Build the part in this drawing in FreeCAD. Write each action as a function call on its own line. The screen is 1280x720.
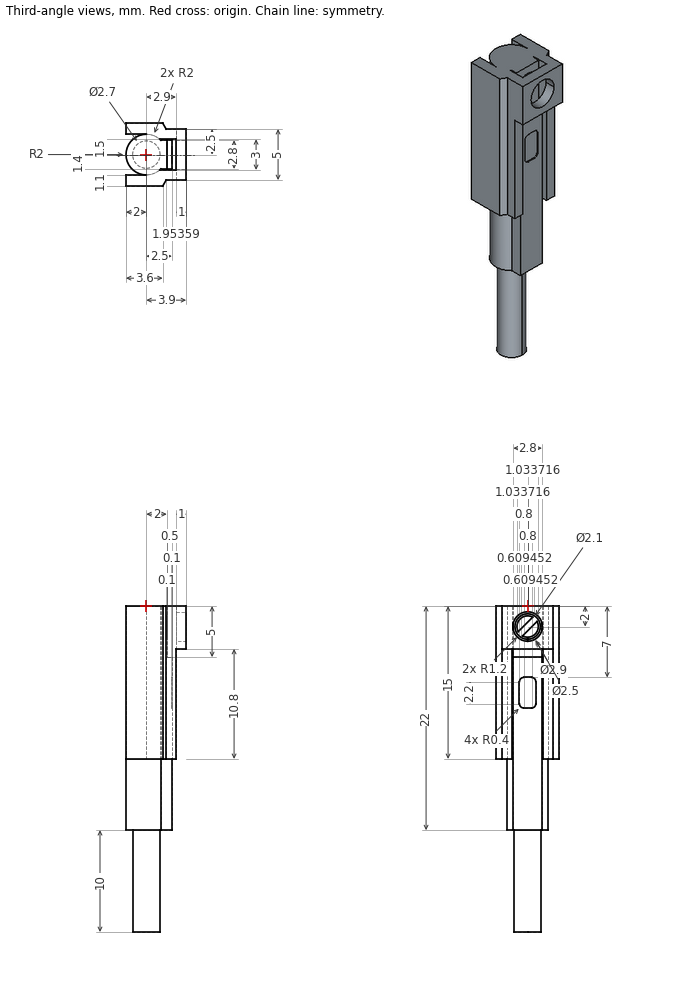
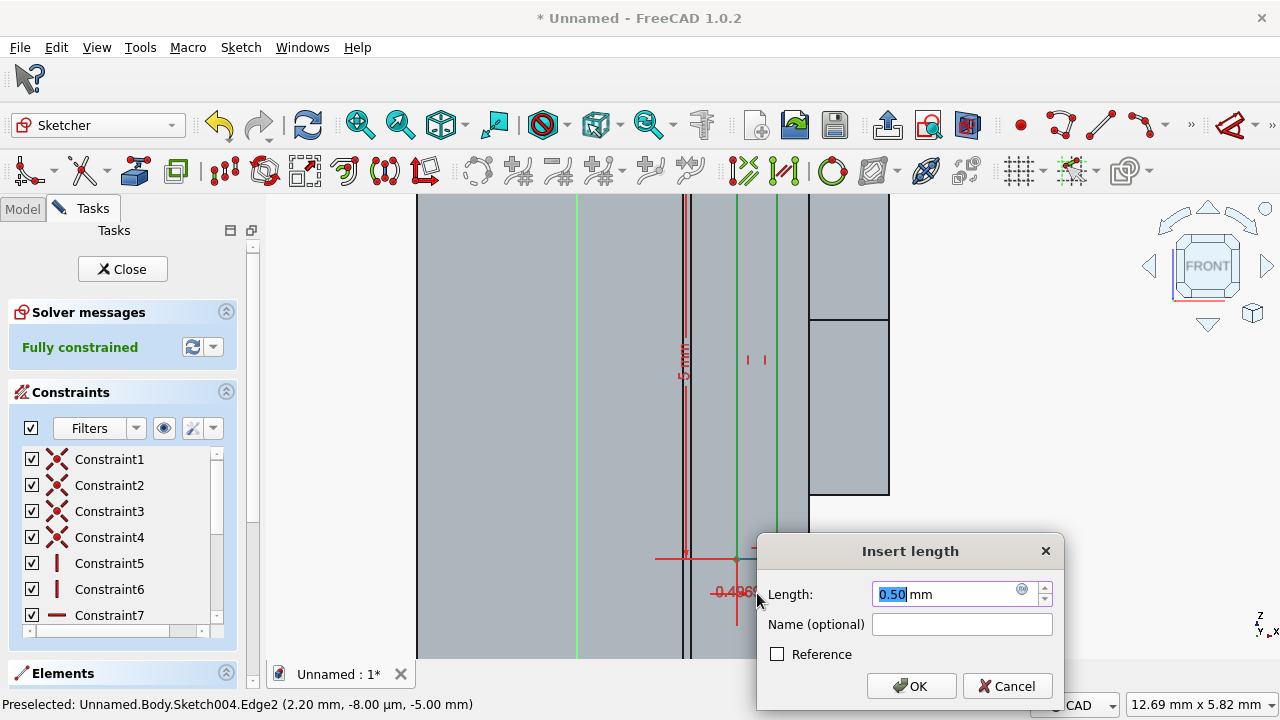
text(0.5)
key(Return)
key(Escape)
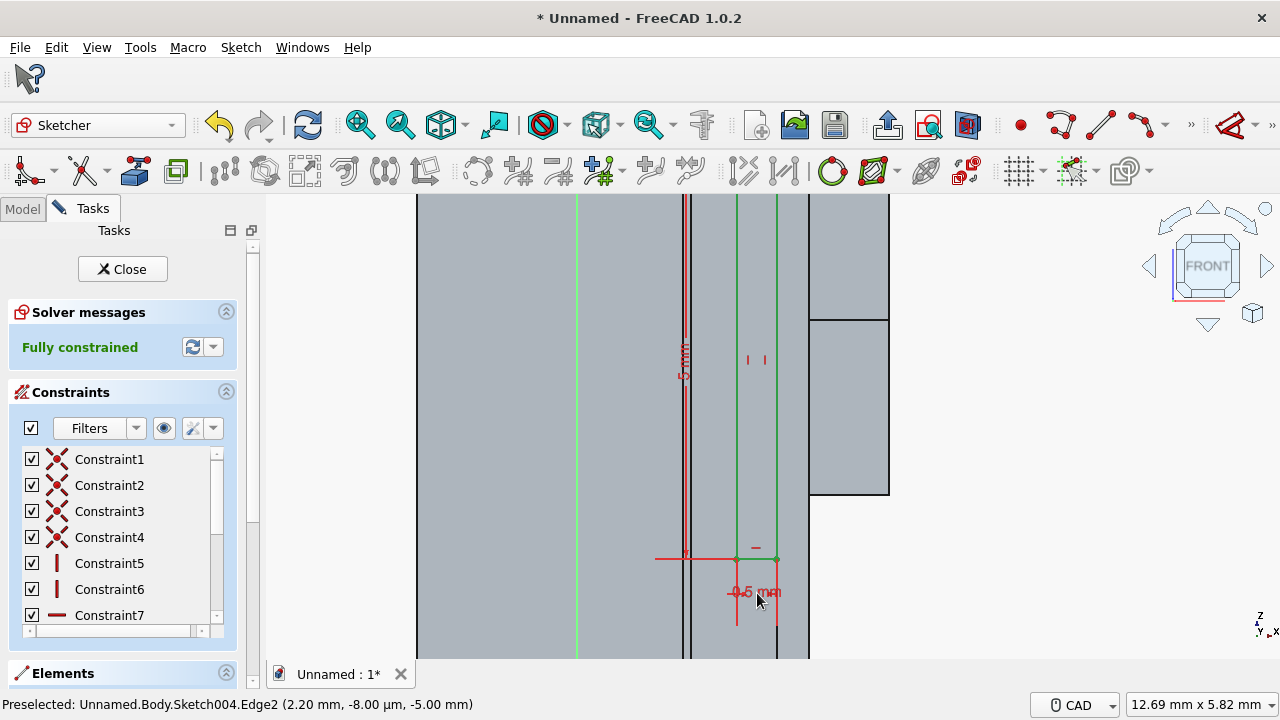
click(123, 269)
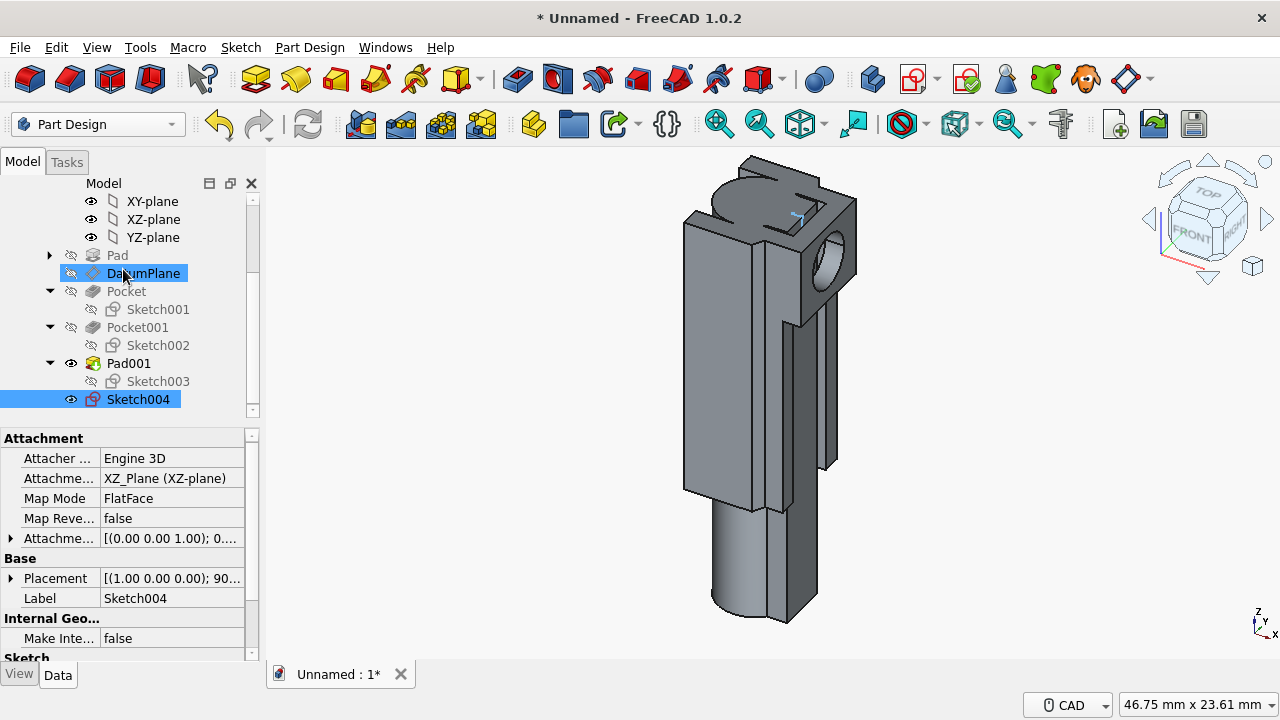
click(518, 80)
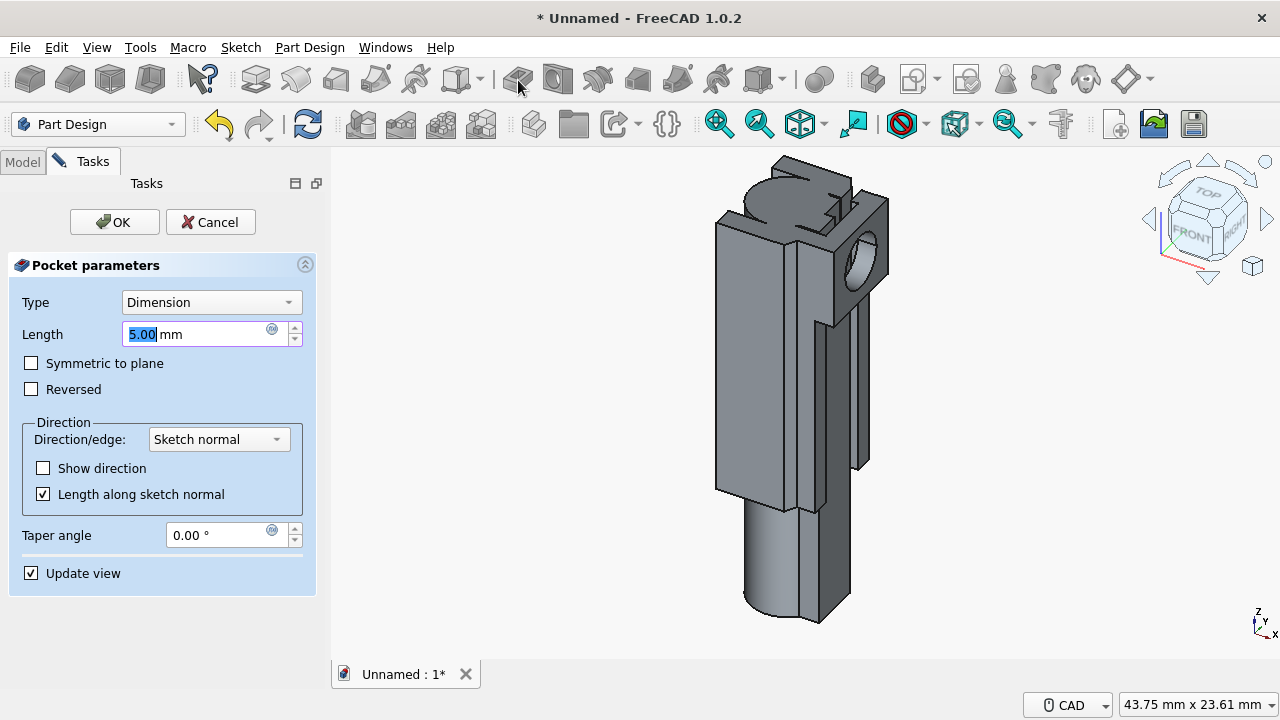
text(2.8)
key(Tab)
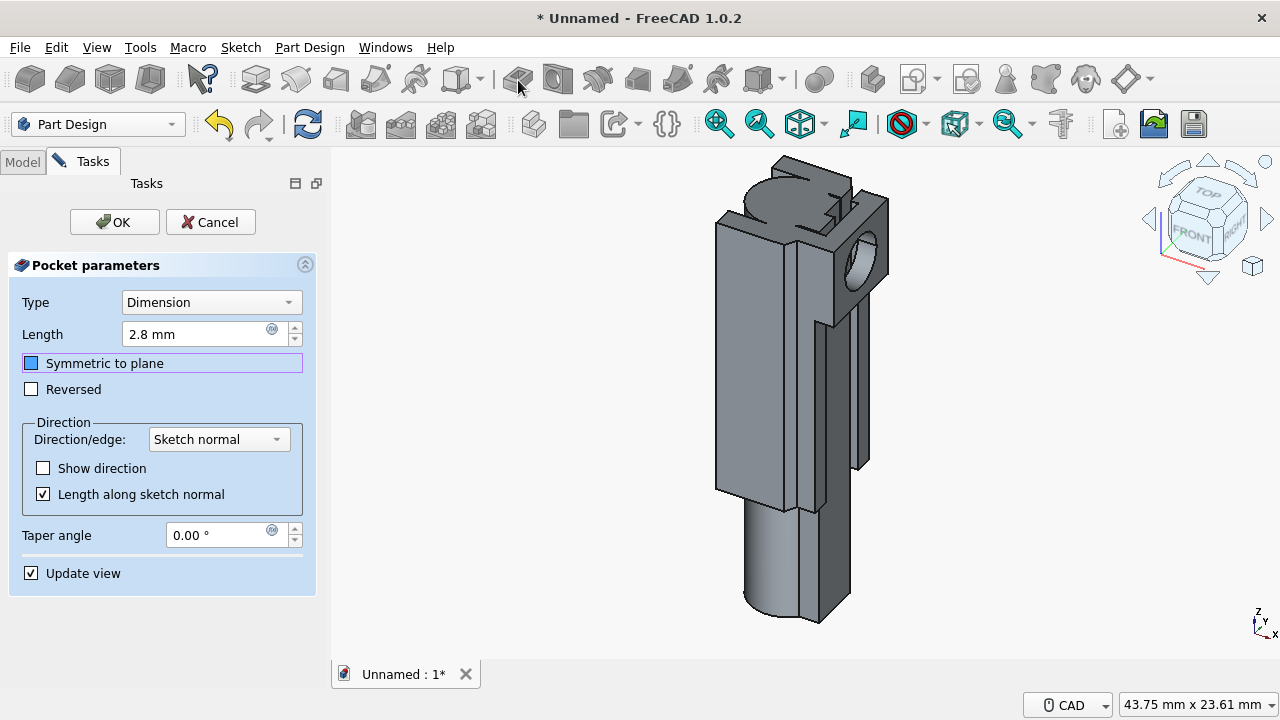
click(30, 363)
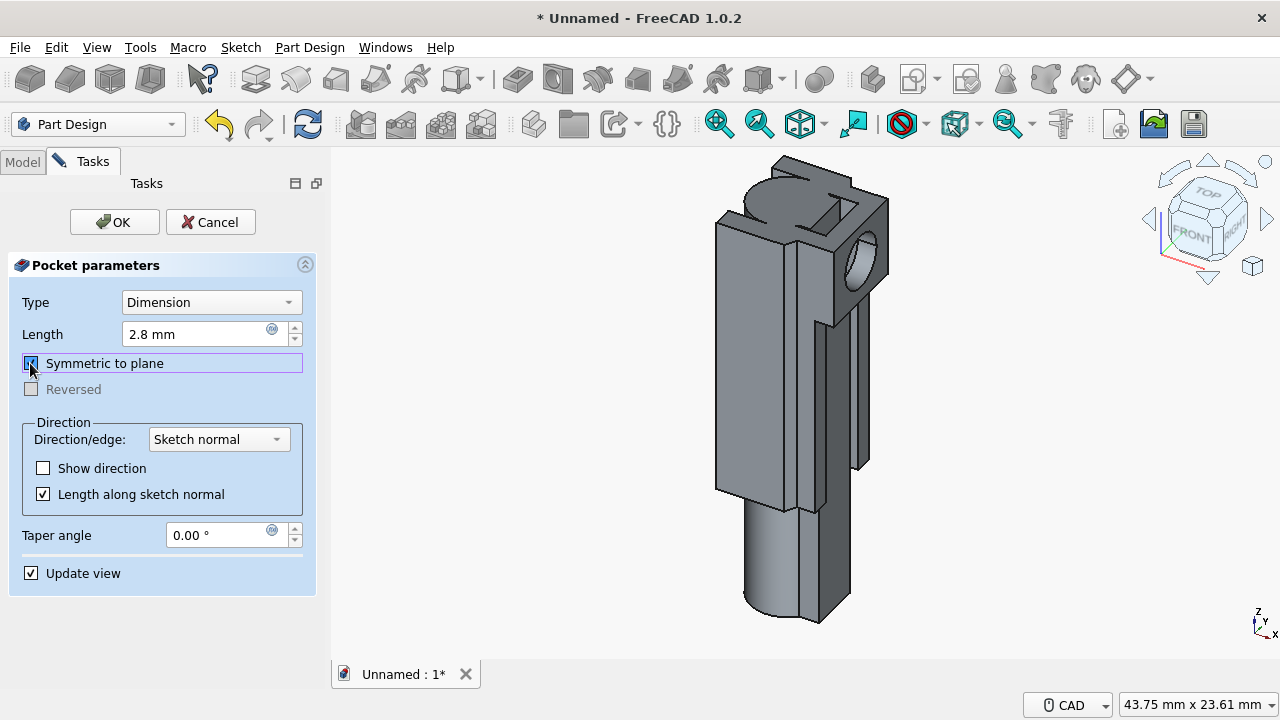
click(115, 222)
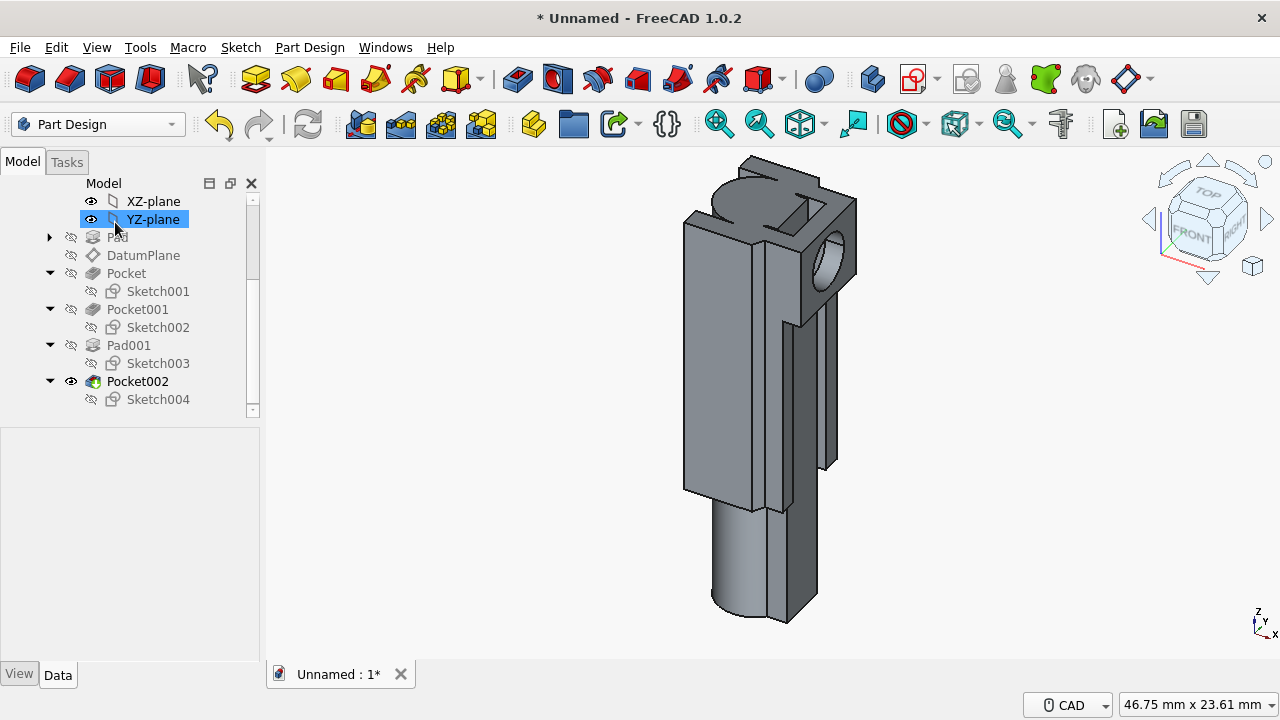
key(0)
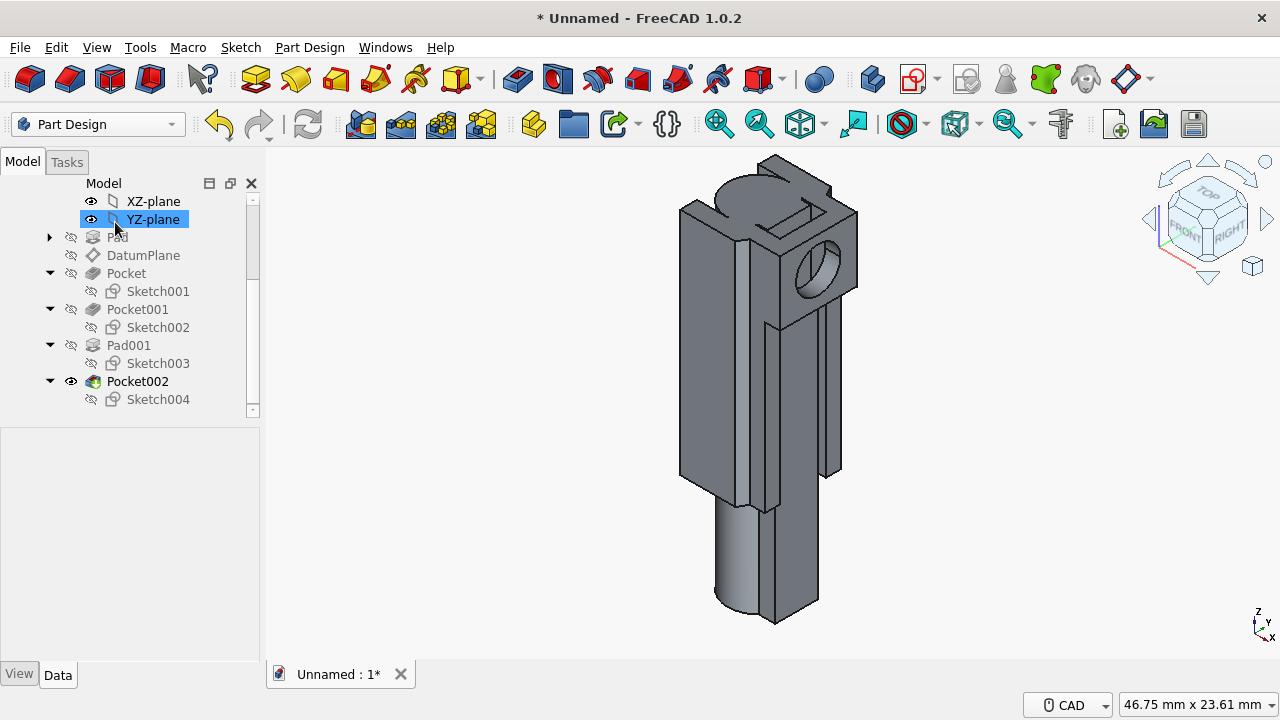
key(3)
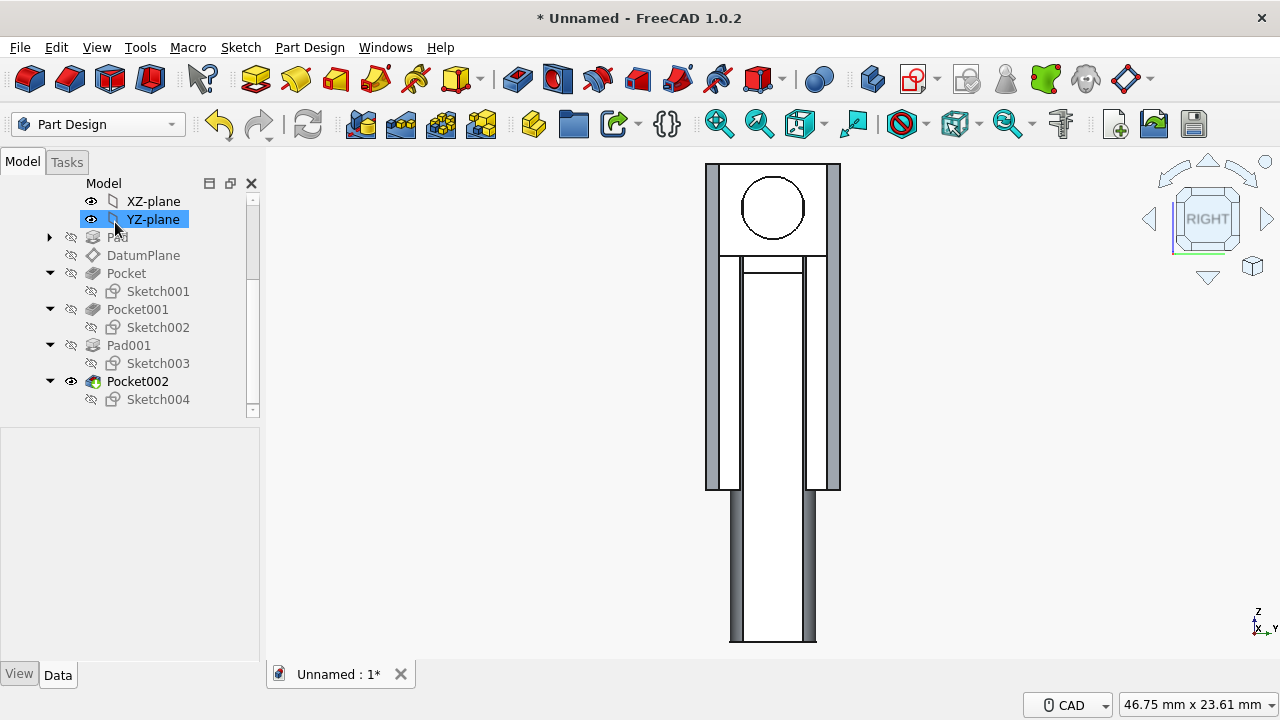
click(773, 202)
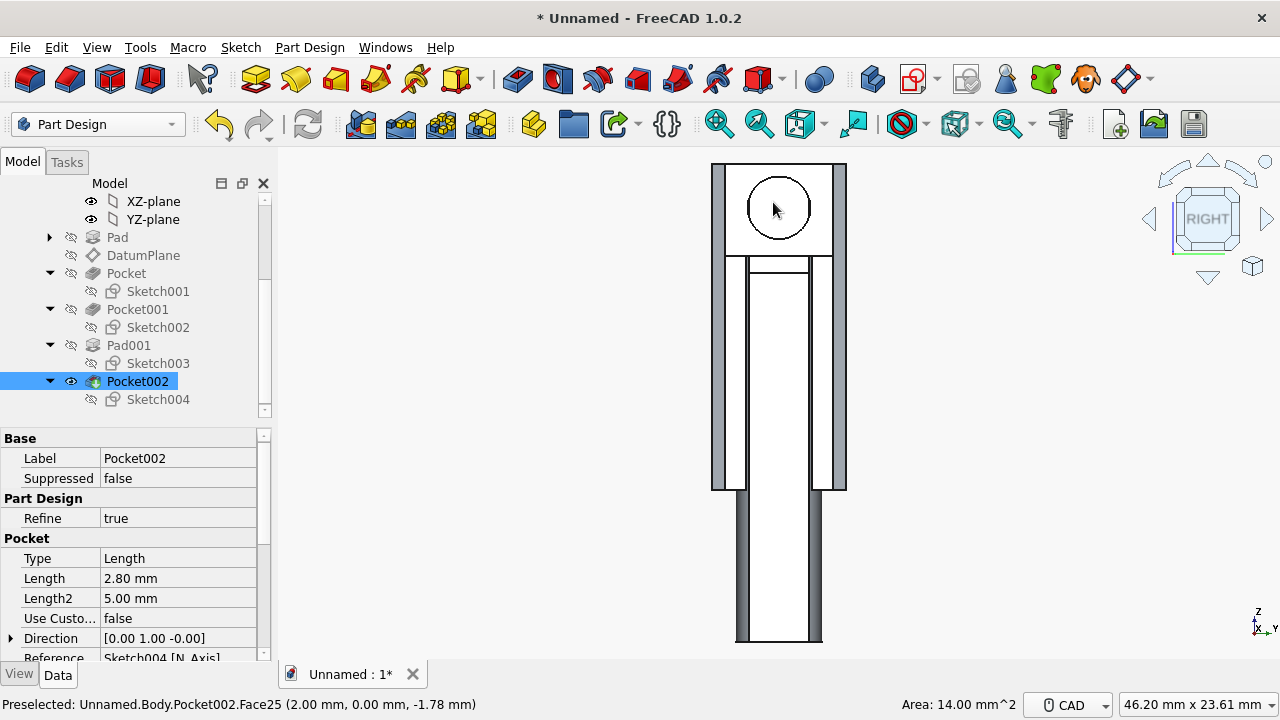
click(914, 80)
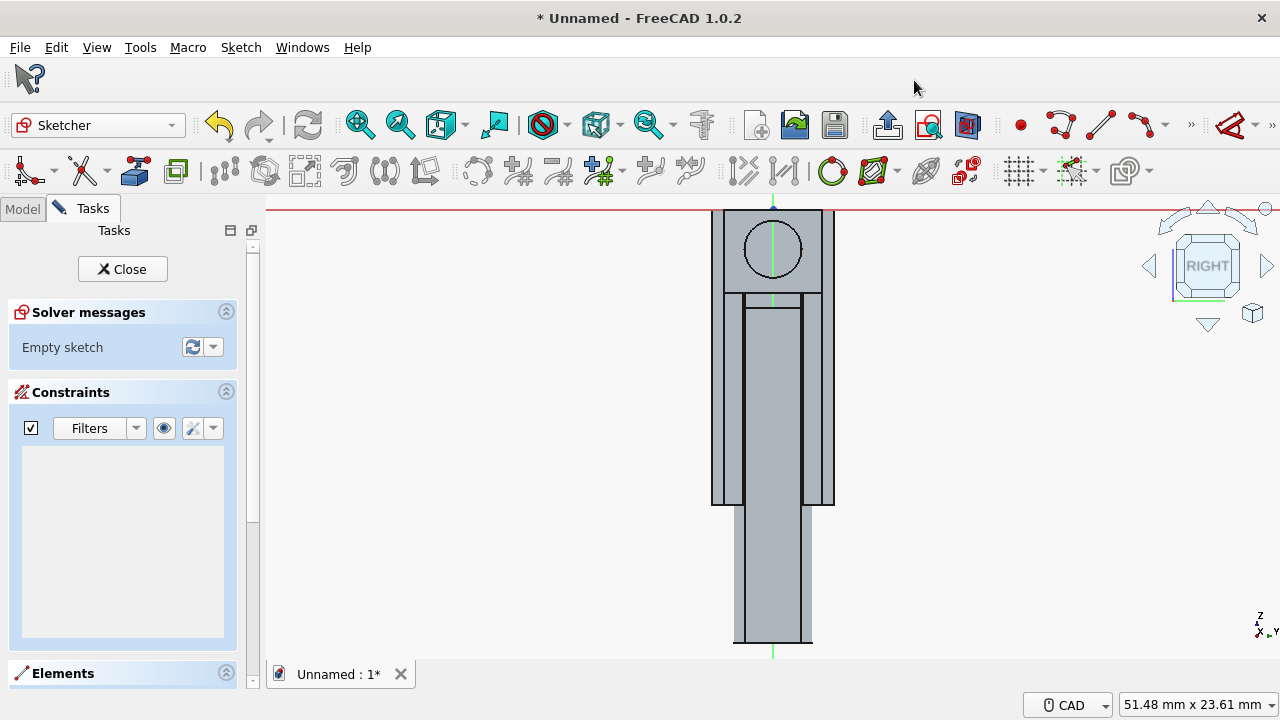
scroll(704, 426, down, 5)